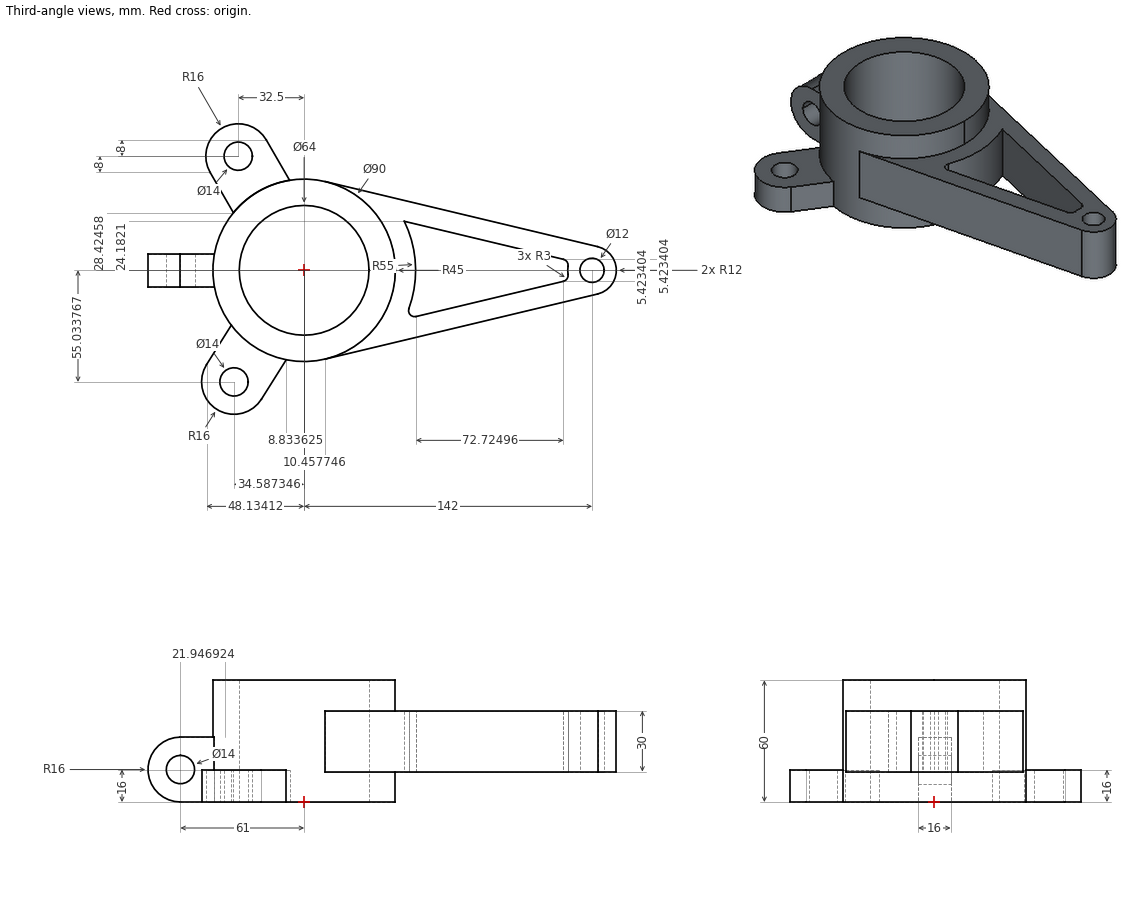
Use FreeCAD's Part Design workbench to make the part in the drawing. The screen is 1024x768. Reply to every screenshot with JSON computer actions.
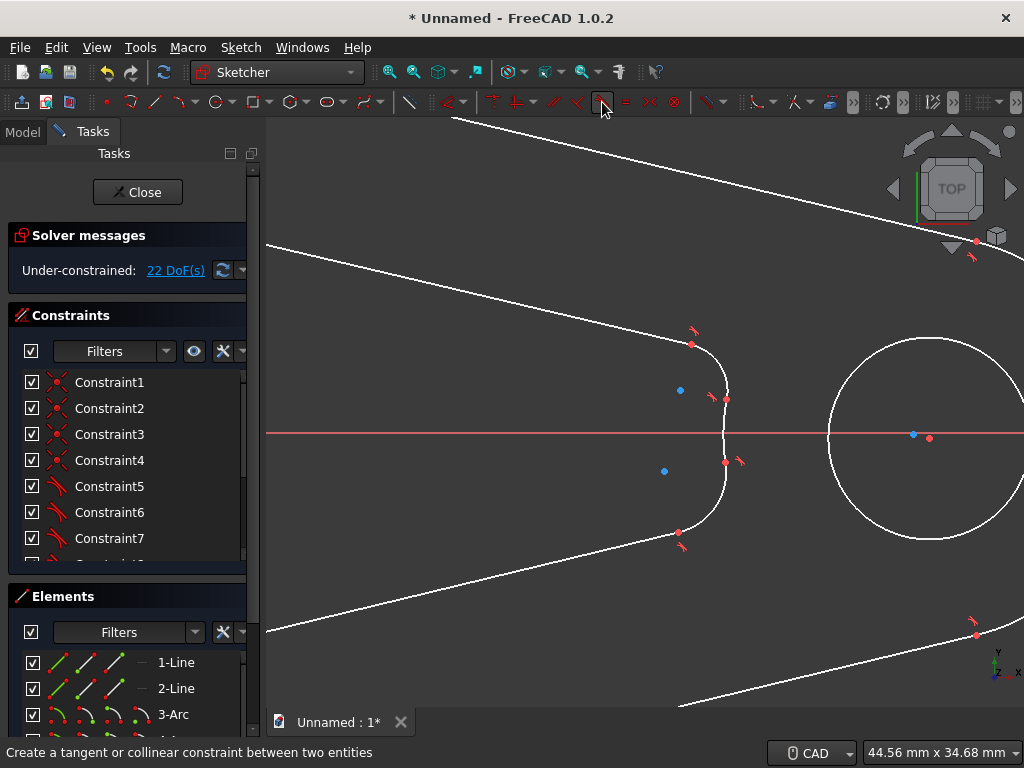
{"action": "scroll", "coordinate": [726, 408], "scroll_direction": "down", "scroll_amount": 9}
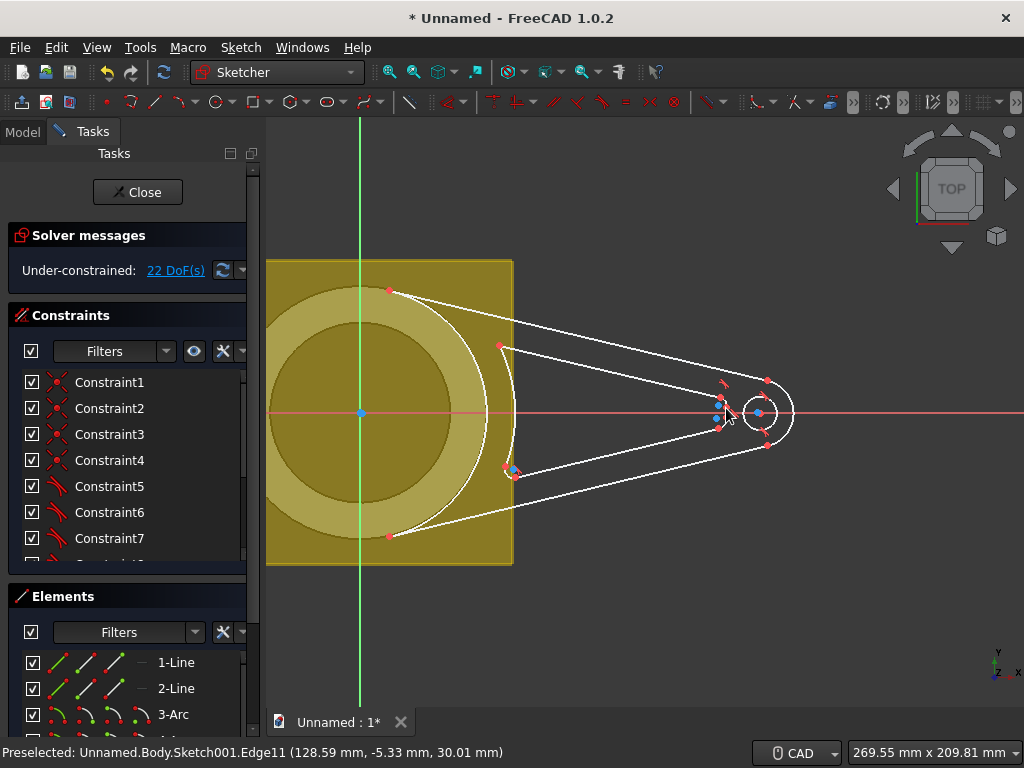
{"action": "left_click", "coordinate": [469, 478]}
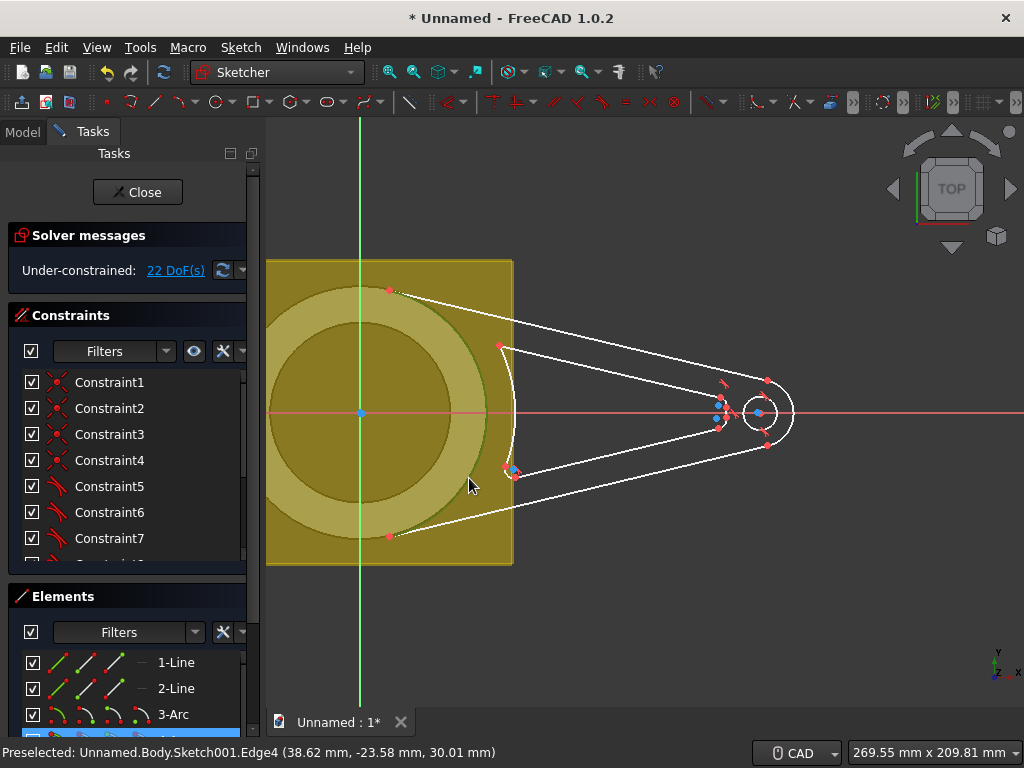
{"action": "left_click", "coordinate": [514, 431]}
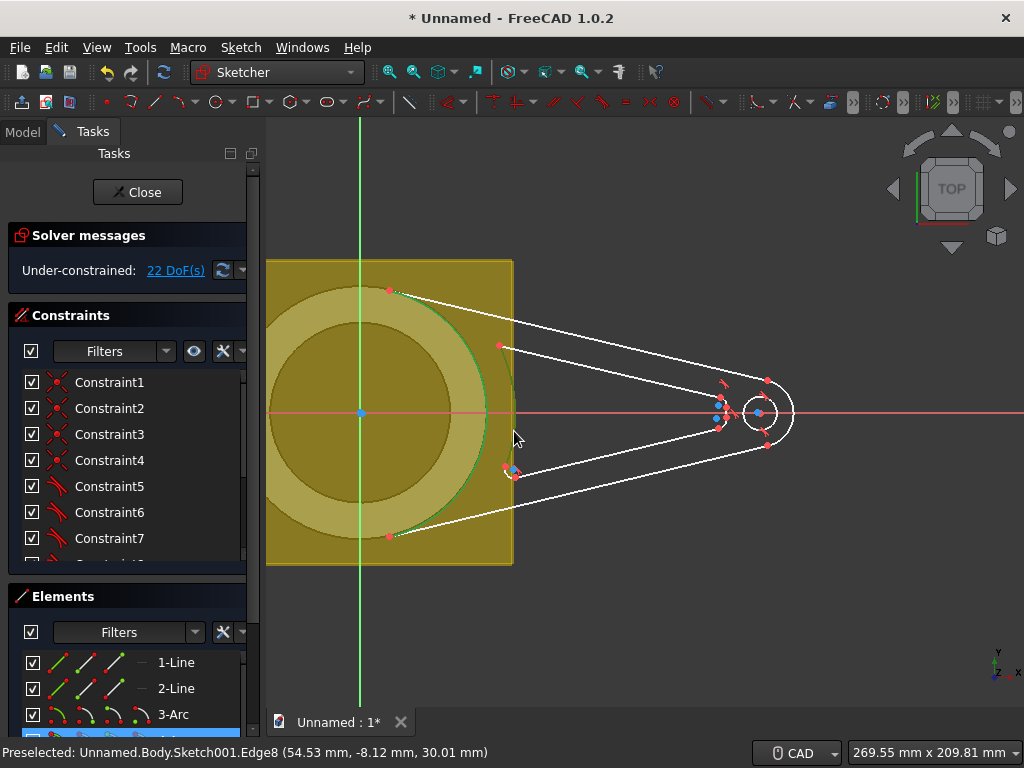
{"action": "left_click", "coordinate": [494, 102]}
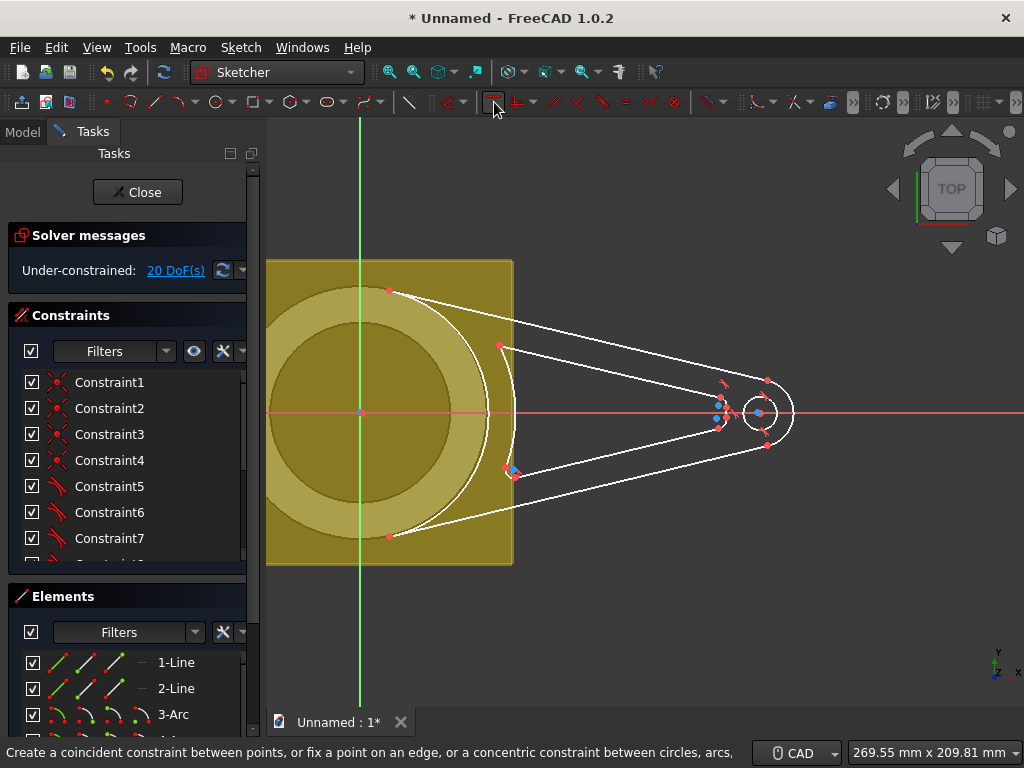
{"action": "scroll", "coordinate": [772, 402], "scroll_direction": "up", "scroll_amount": 2}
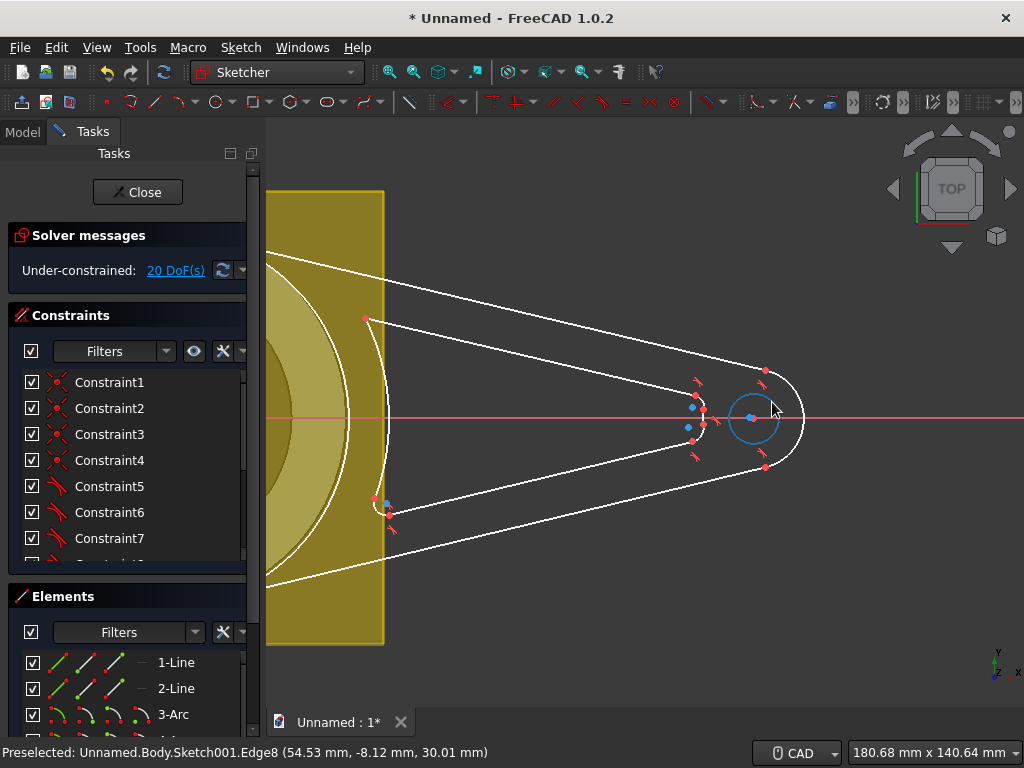
{"action": "left_click", "coordinate": [772, 401]}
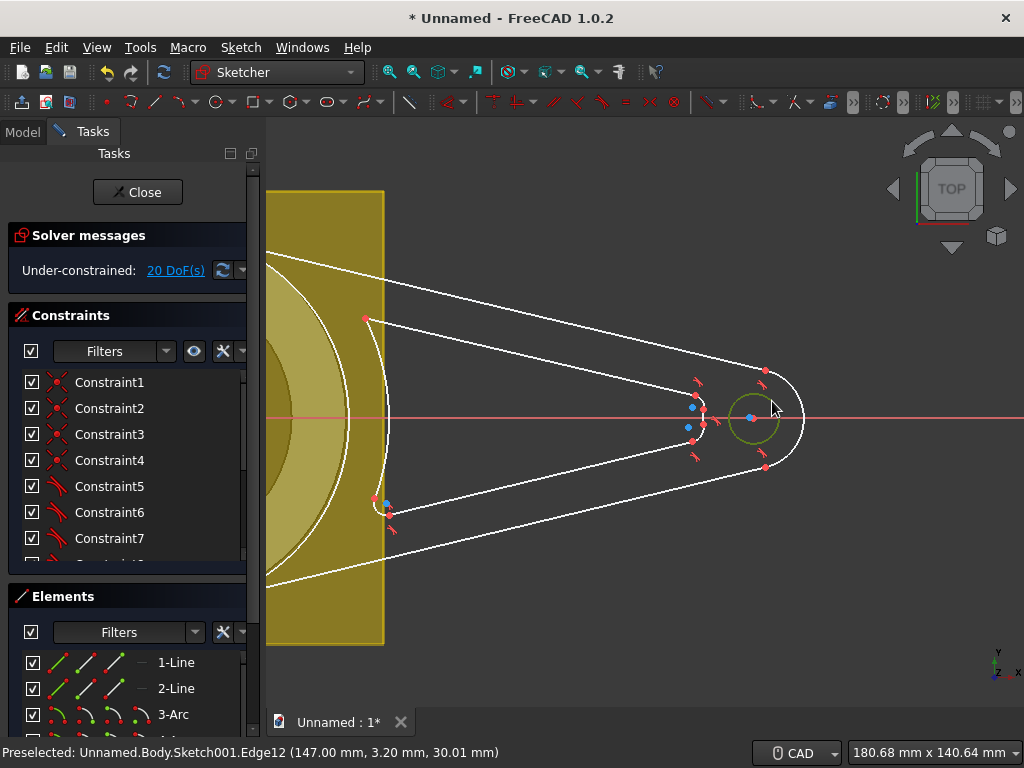
{"action": "scroll", "coordinate": [703, 417], "scroll_direction": "up", "scroll_amount": 3}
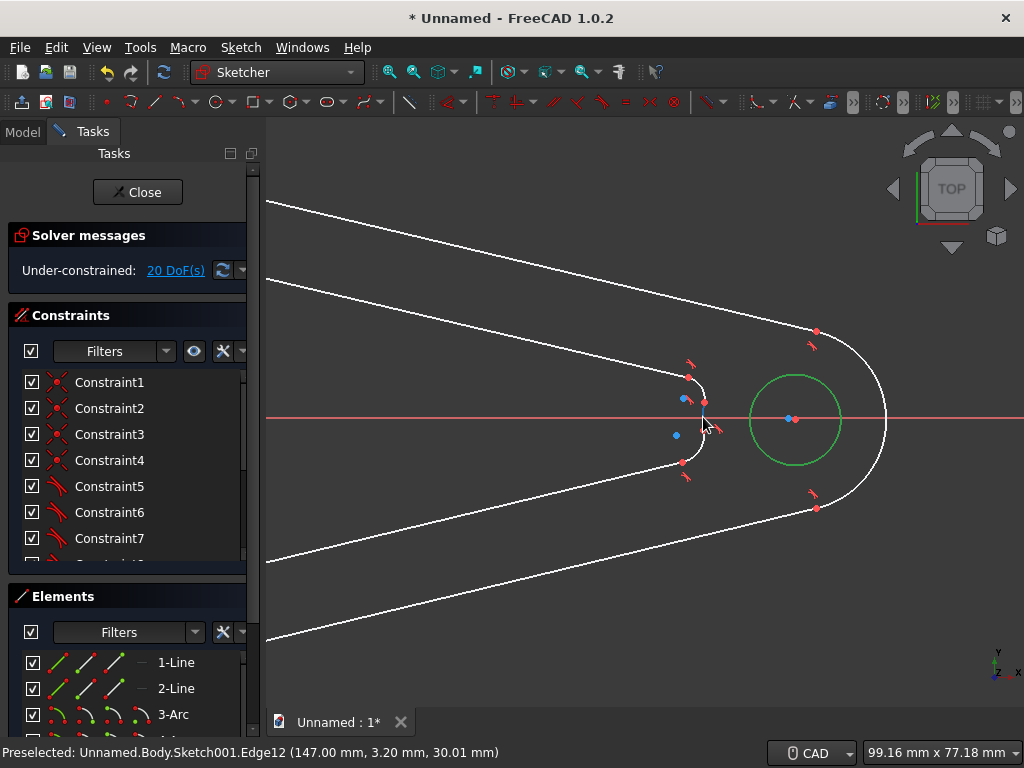
{"action": "left_click", "coordinate": [703, 417]}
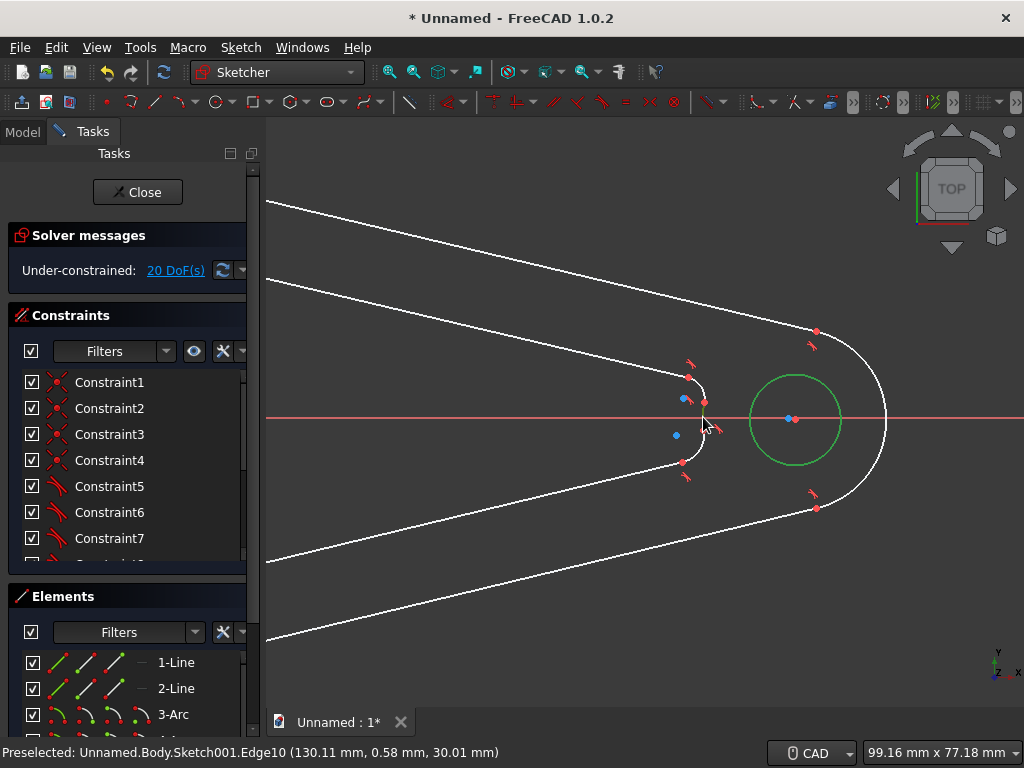
{"action": "key", "text": "c"}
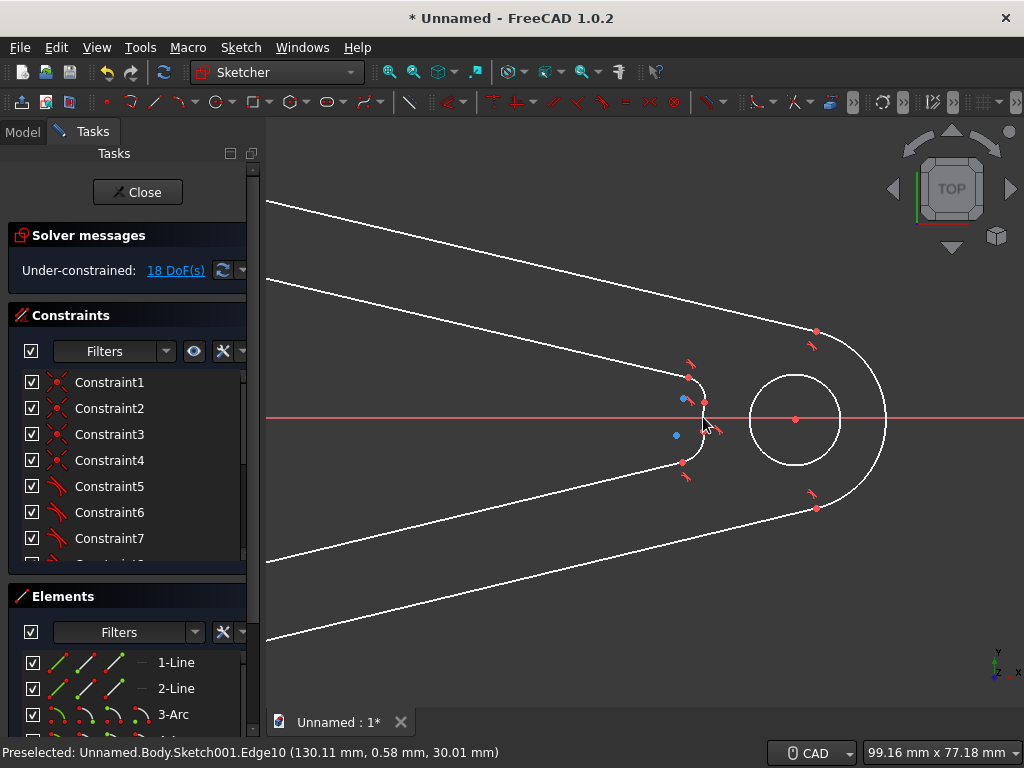
{"action": "scroll", "coordinate": [739, 409], "scroll_direction": "down", "scroll_amount": 5}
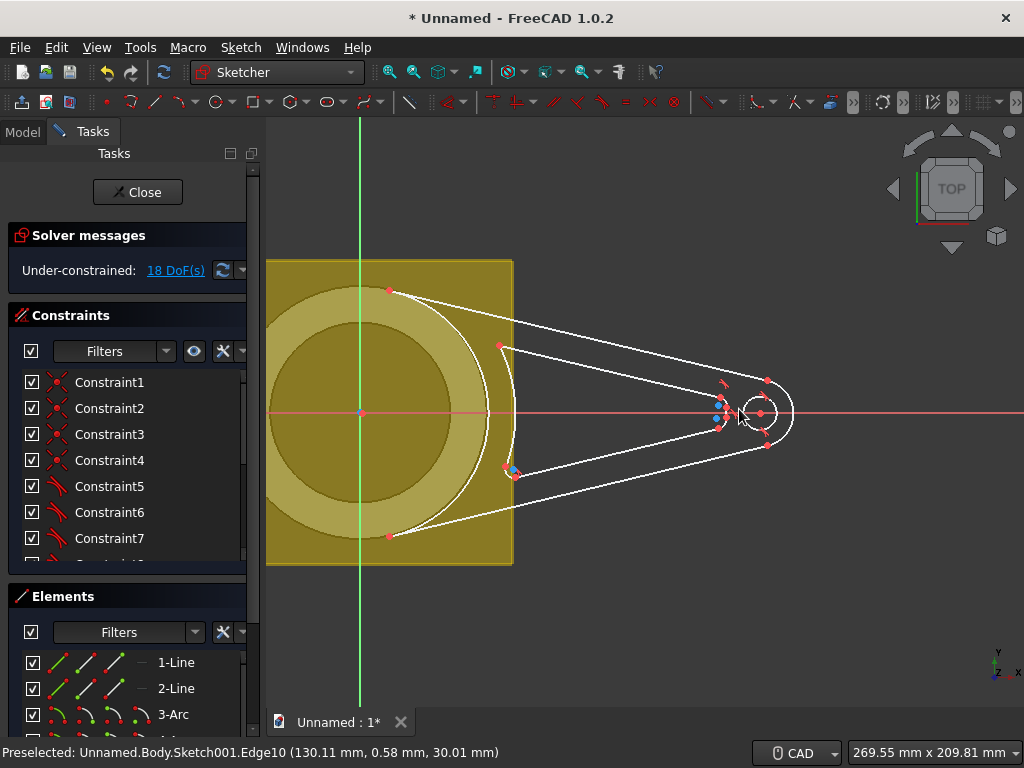
{"action": "scroll", "coordinate": [361, 413], "scroll_direction": "up", "scroll_amount": 9}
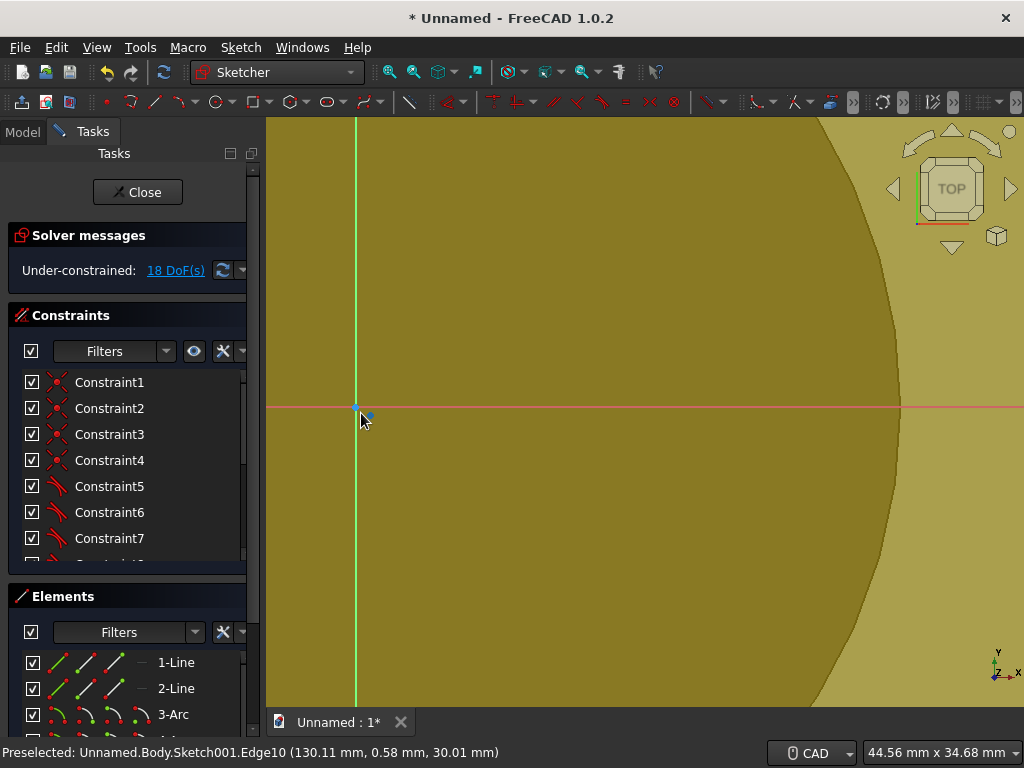
{"action": "left_click_drag", "start_coordinate": [346, 397], "coordinate": [381, 426]}